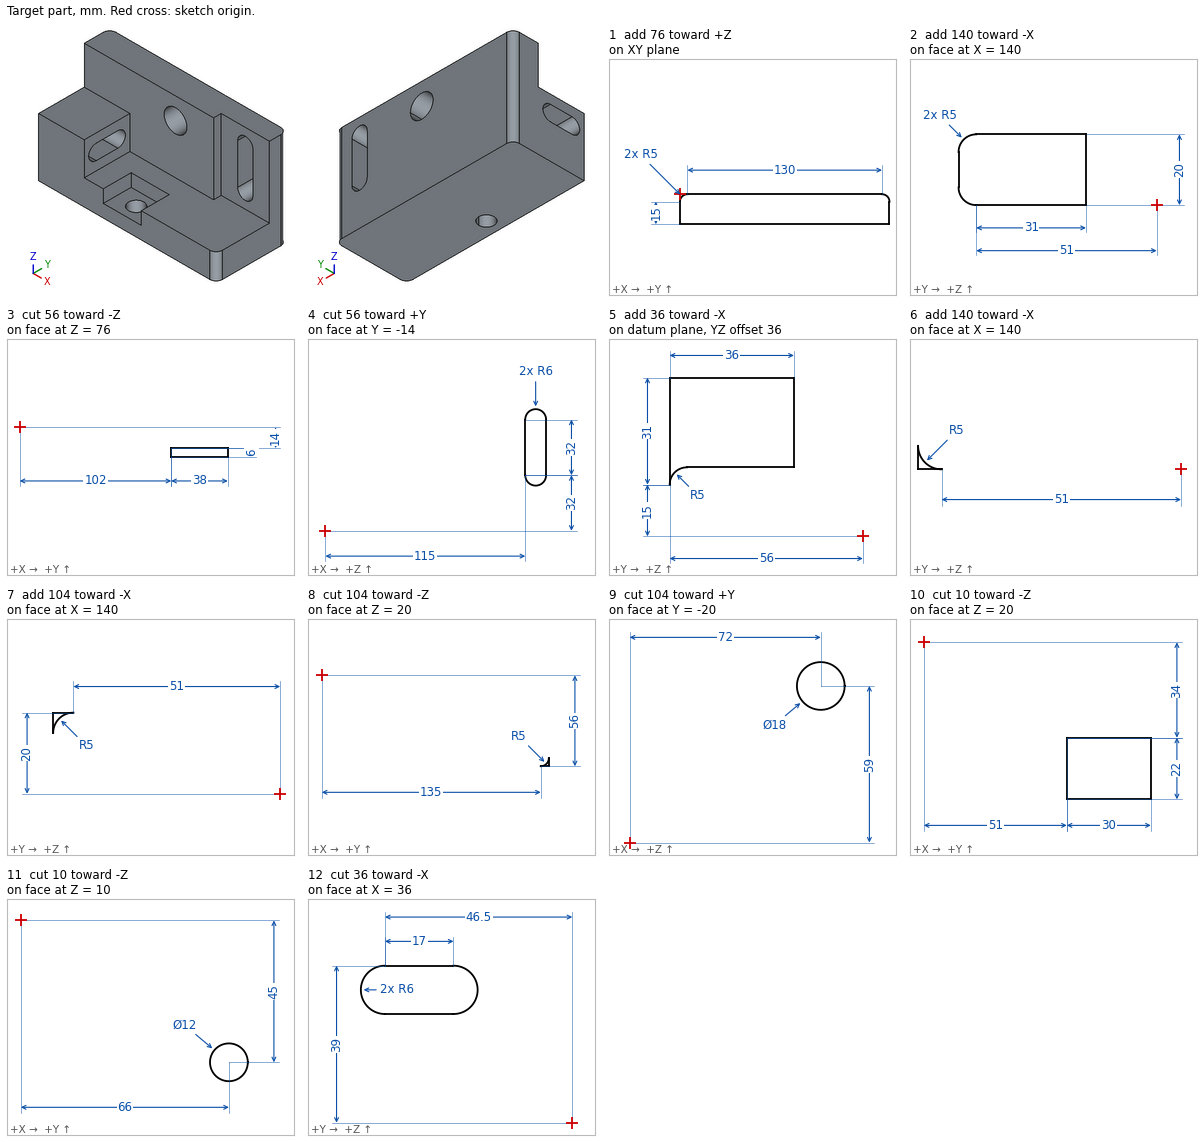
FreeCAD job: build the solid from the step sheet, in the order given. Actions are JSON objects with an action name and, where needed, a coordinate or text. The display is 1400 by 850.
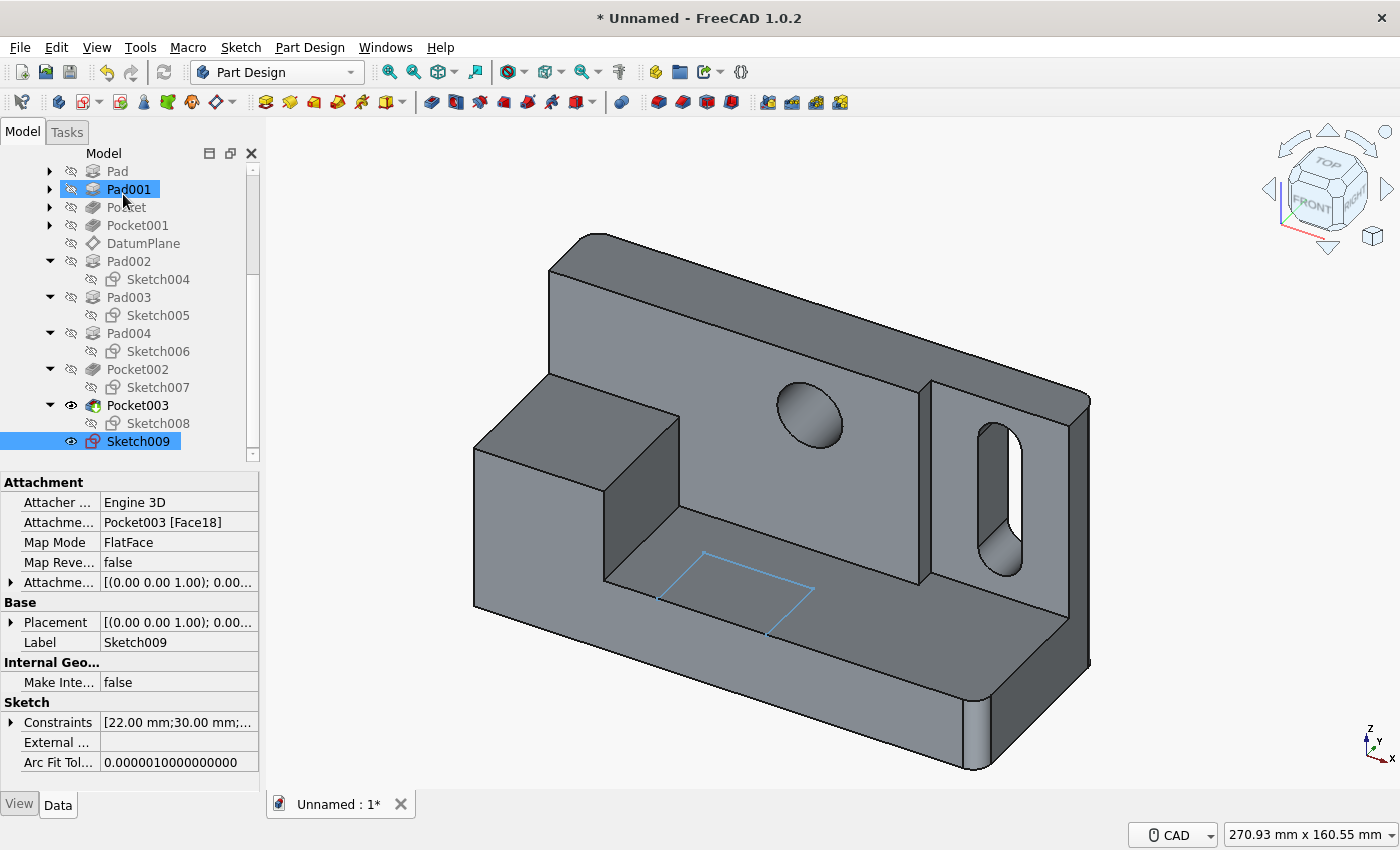
{"action": "left_click", "coordinate": [432, 102]}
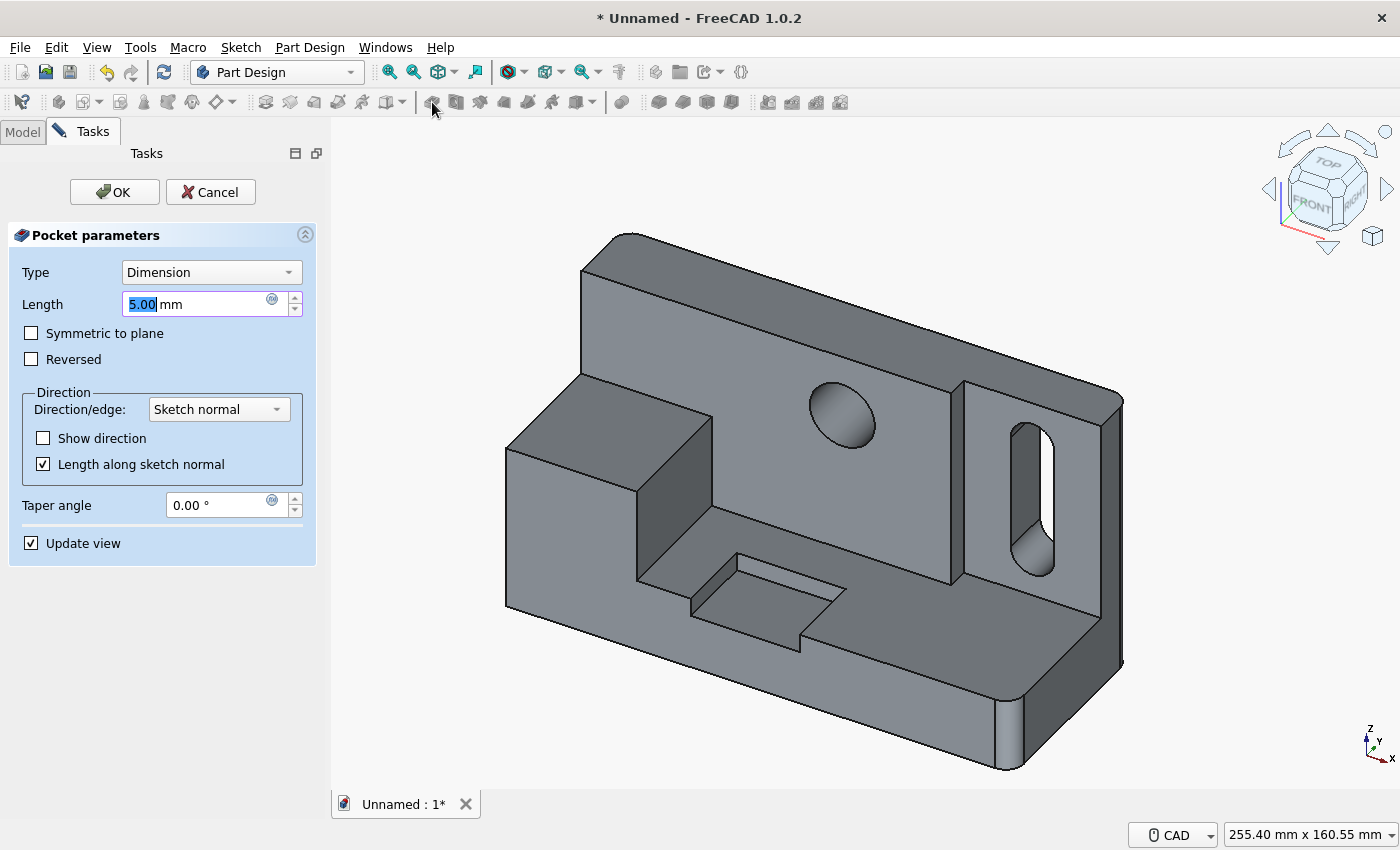
{"action": "type", "text": "10"}
{"action": "key", "text": "Tab"}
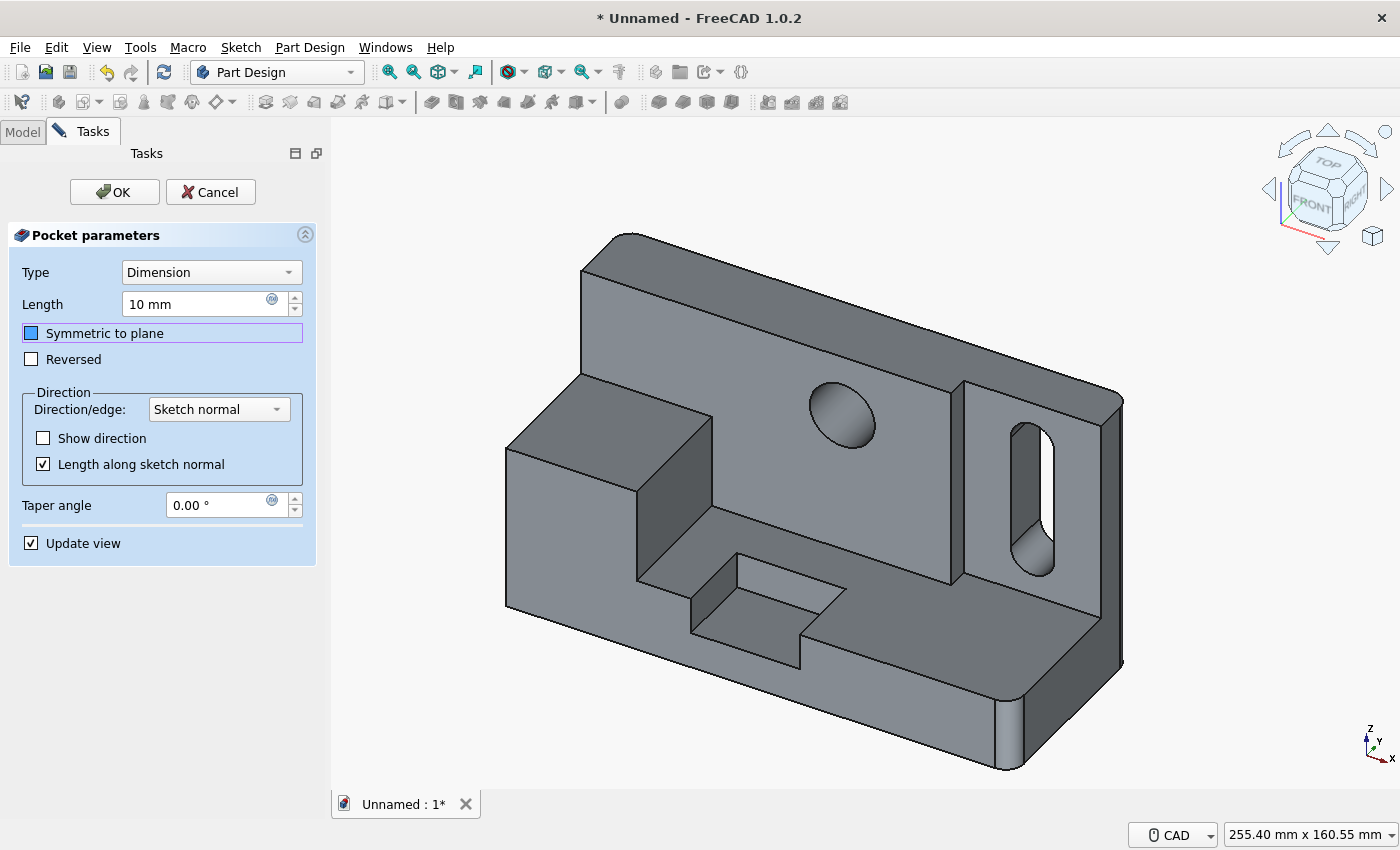
{"action": "left_click", "coordinate": [115, 192]}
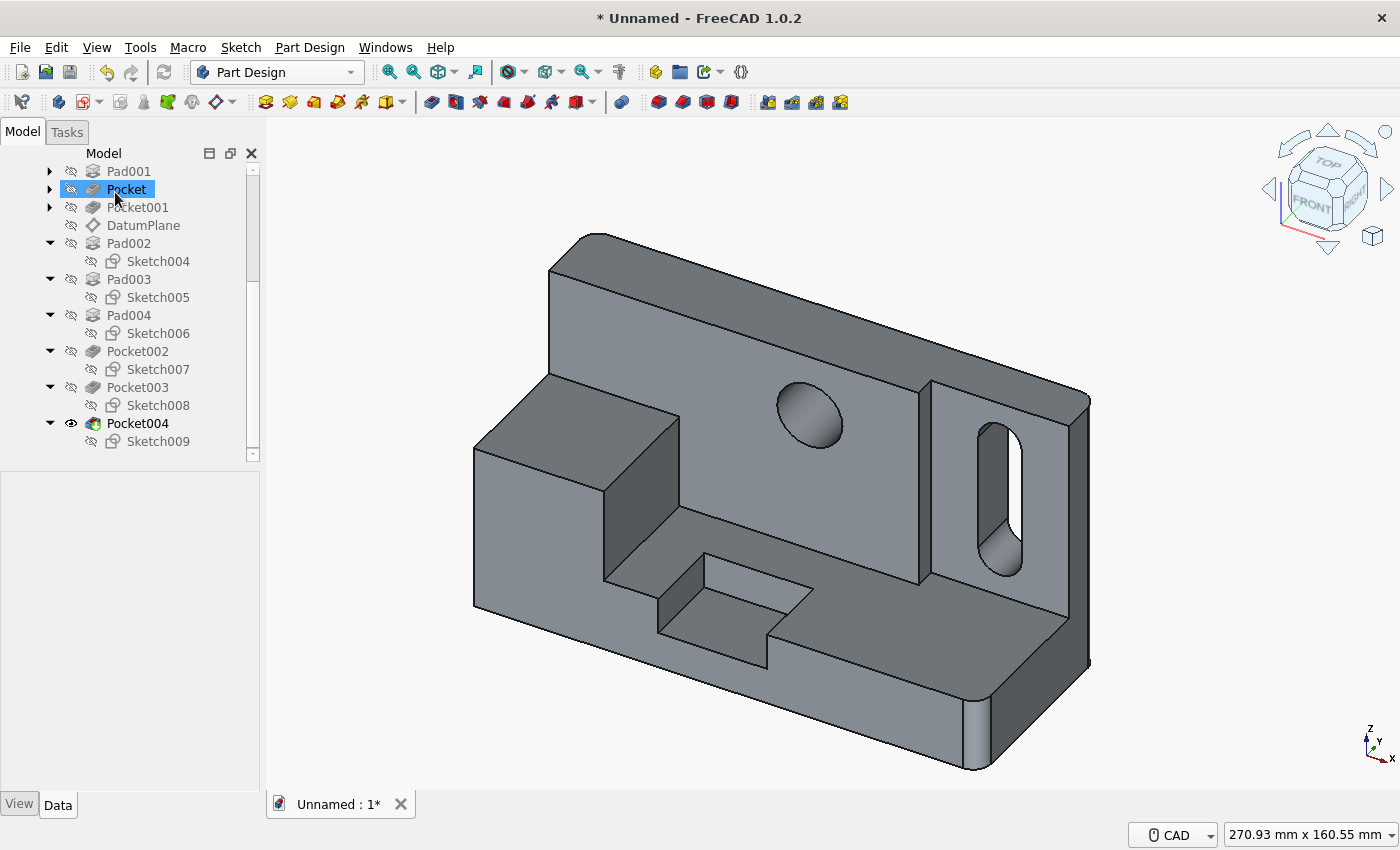
{"action": "left_click", "coordinate": [736, 627]}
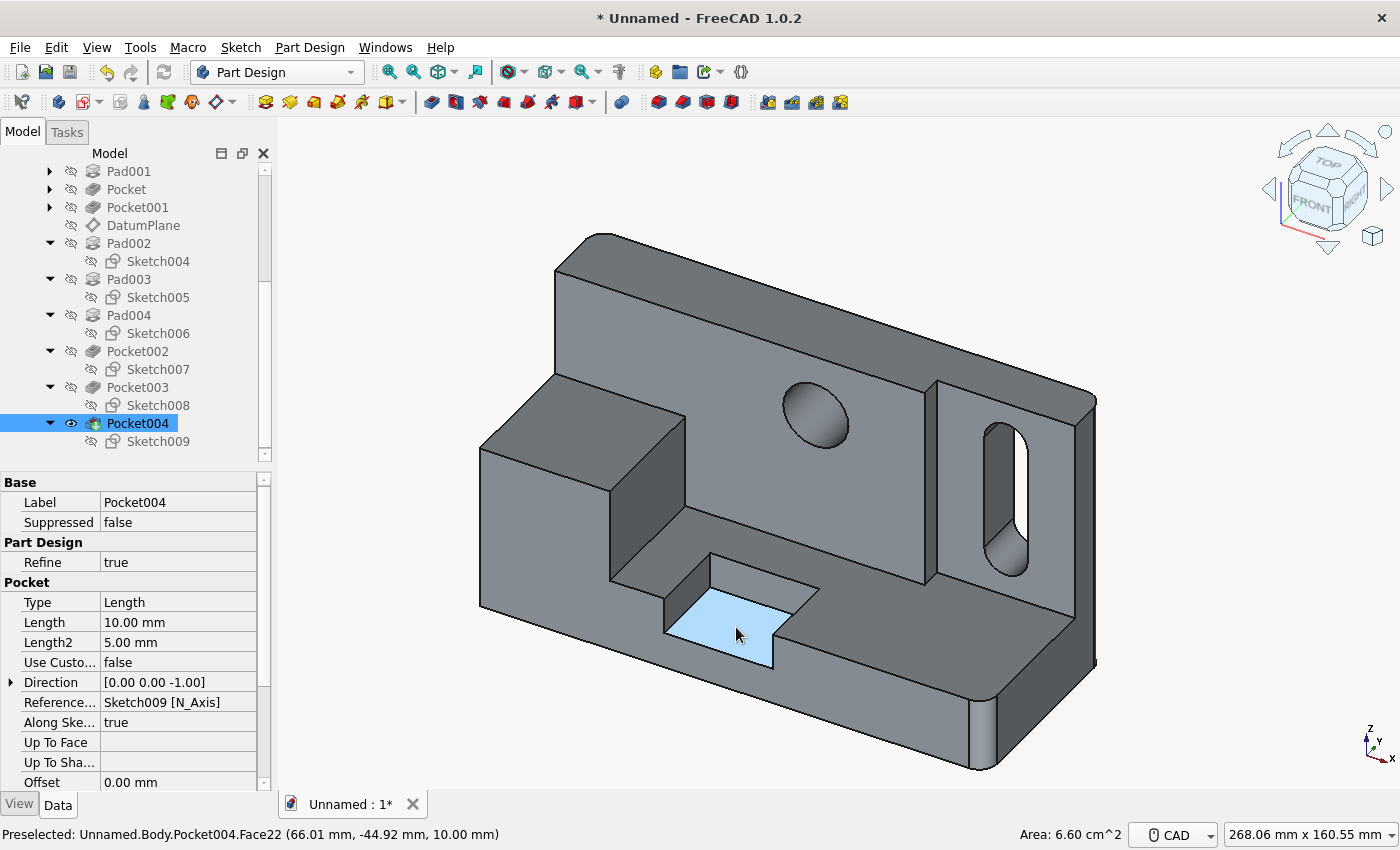
{"action": "left_click", "coordinate": [84, 102]}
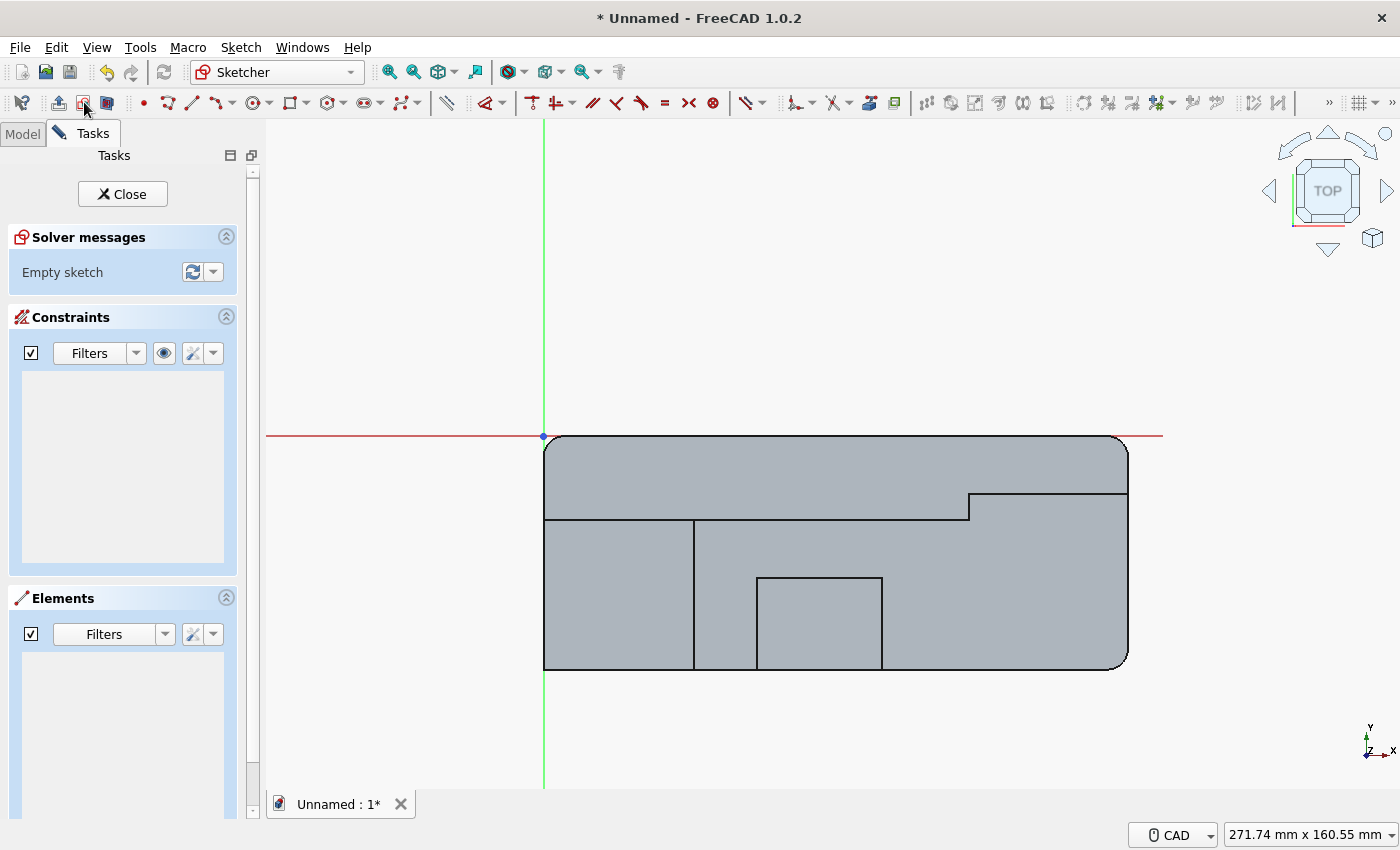
{"action": "left_click", "coordinate": [108, 104]}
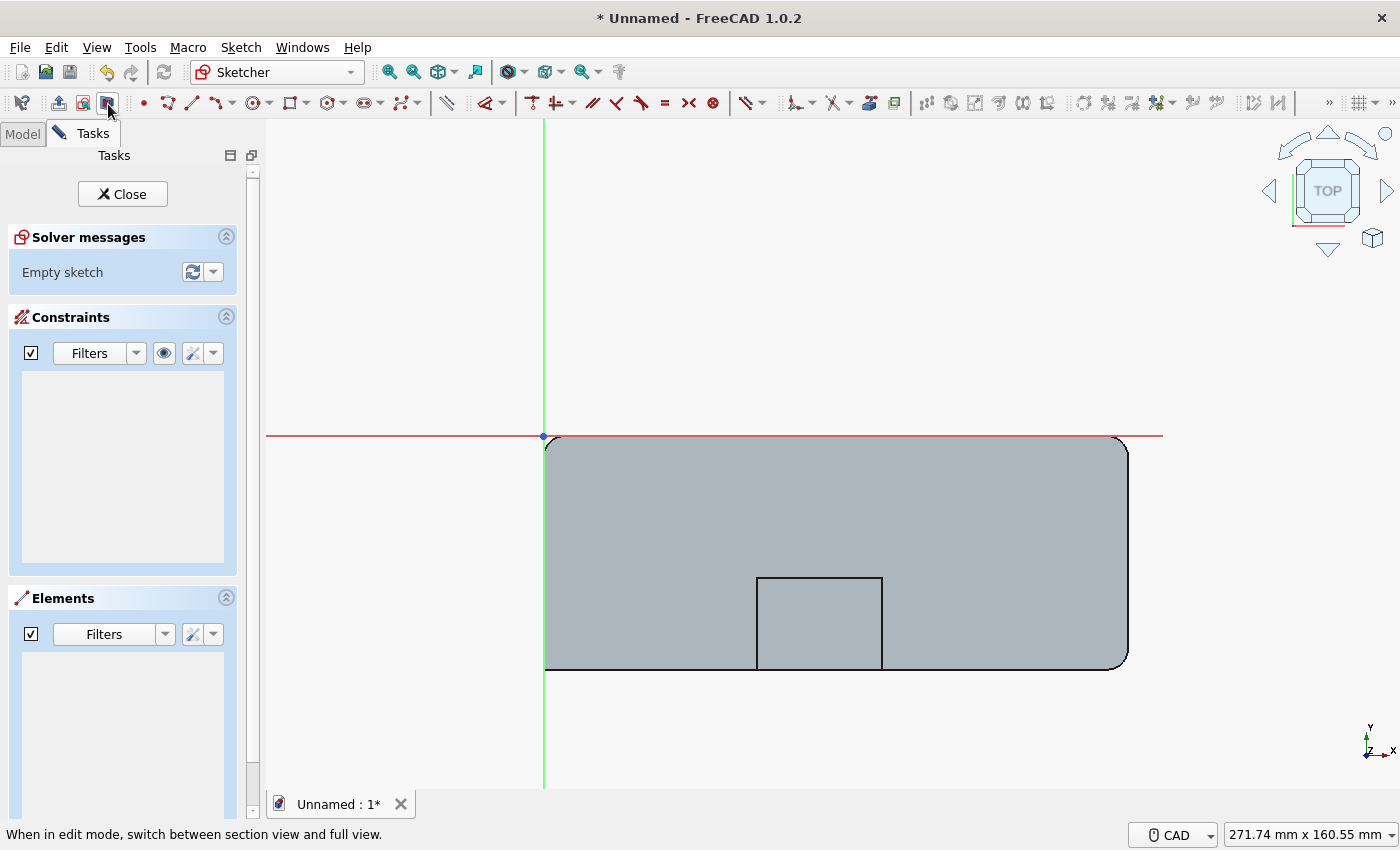
{"action": "scroll", "coordinate": [826, 645], "scroll_direction": "up", "scroll_amount": 11}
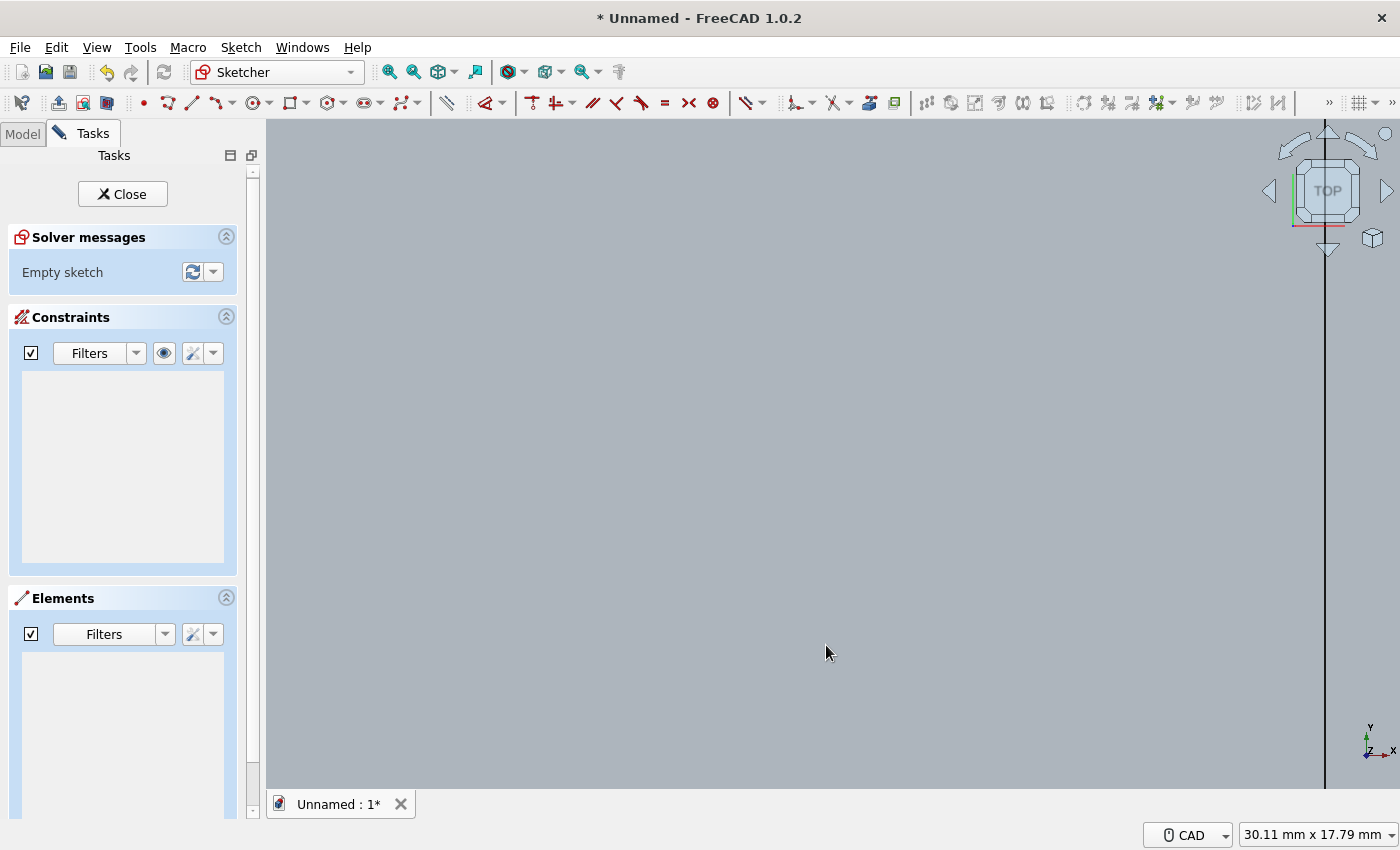
{"action": "left_click", "coordinate": [254, 104]}